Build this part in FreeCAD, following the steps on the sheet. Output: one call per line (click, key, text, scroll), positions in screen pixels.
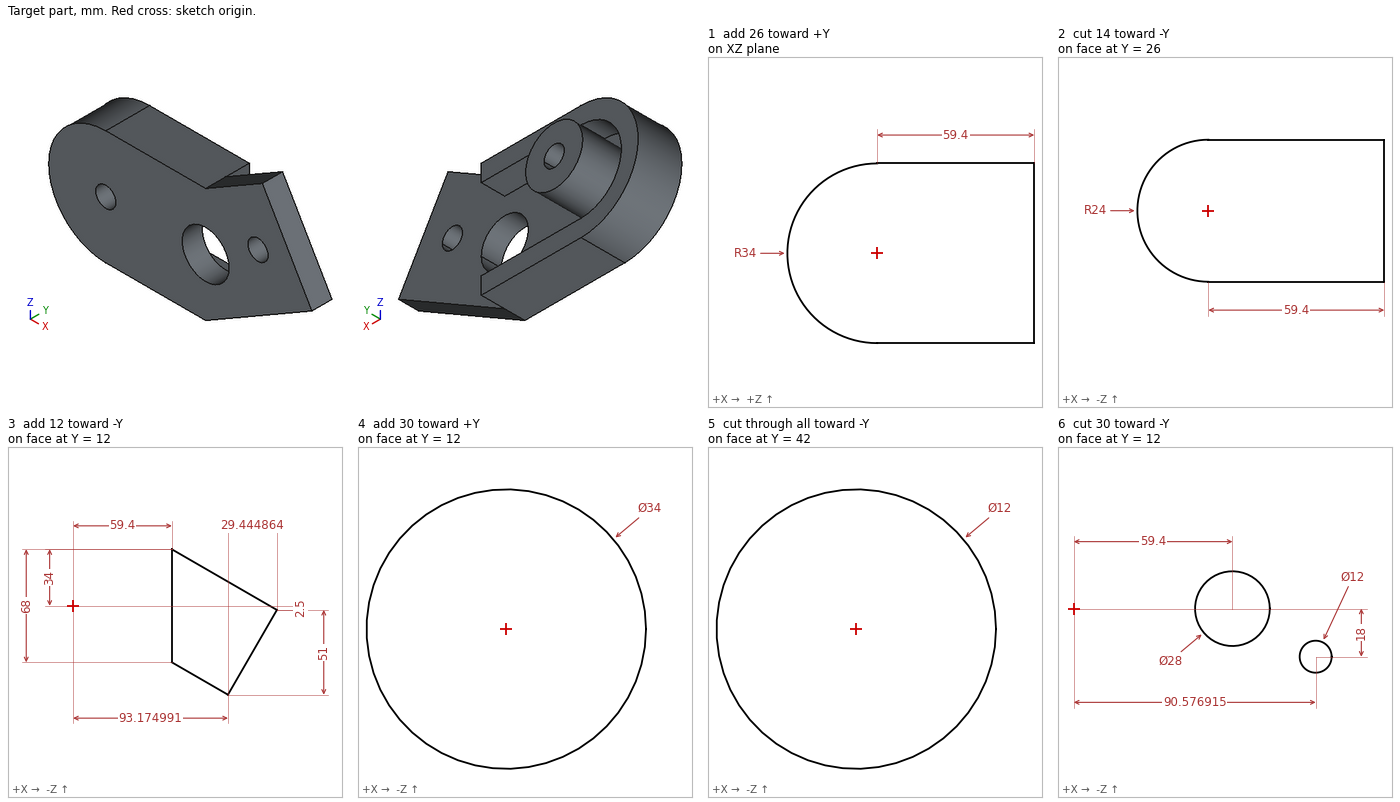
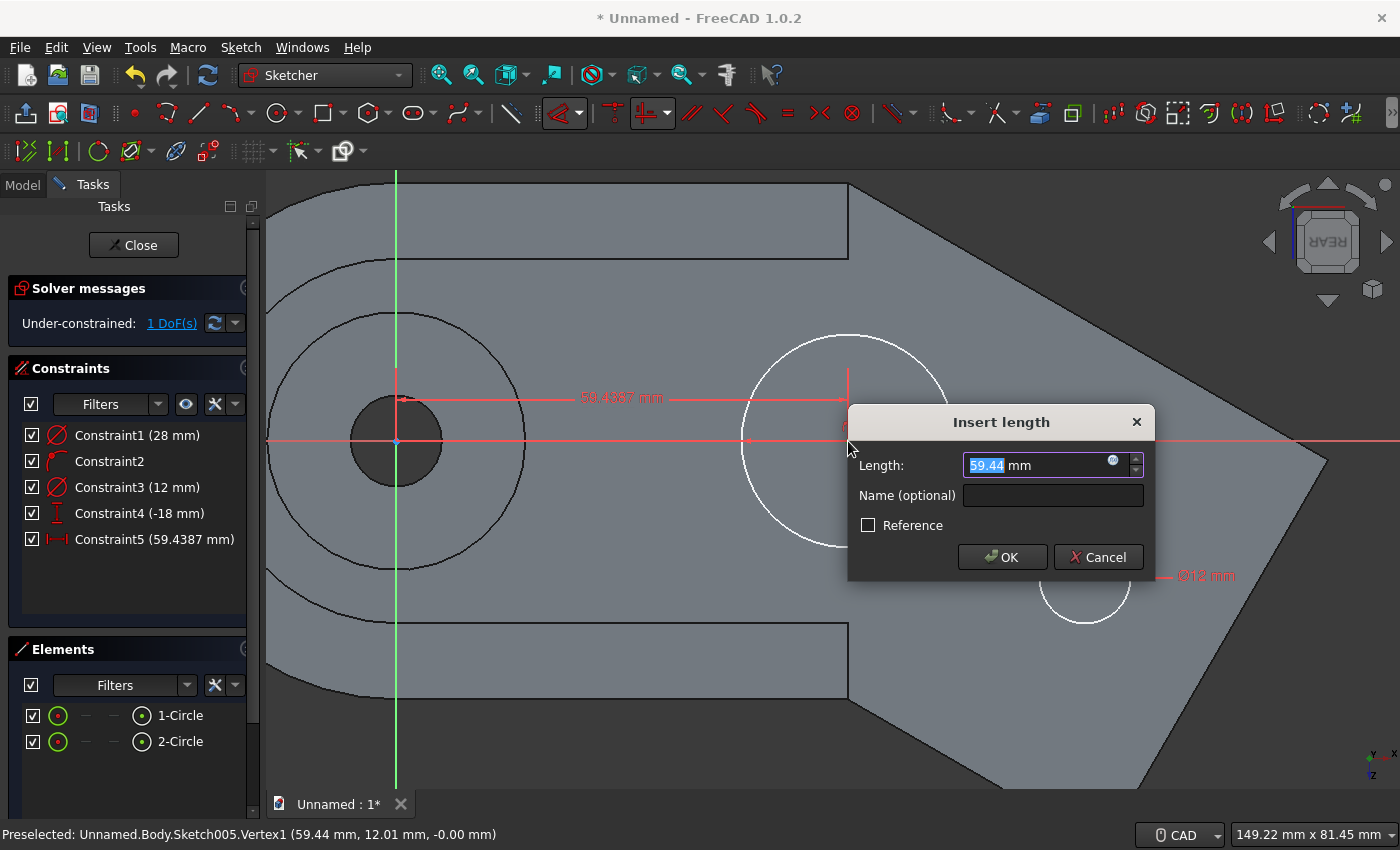
text(59.4)
key(Return)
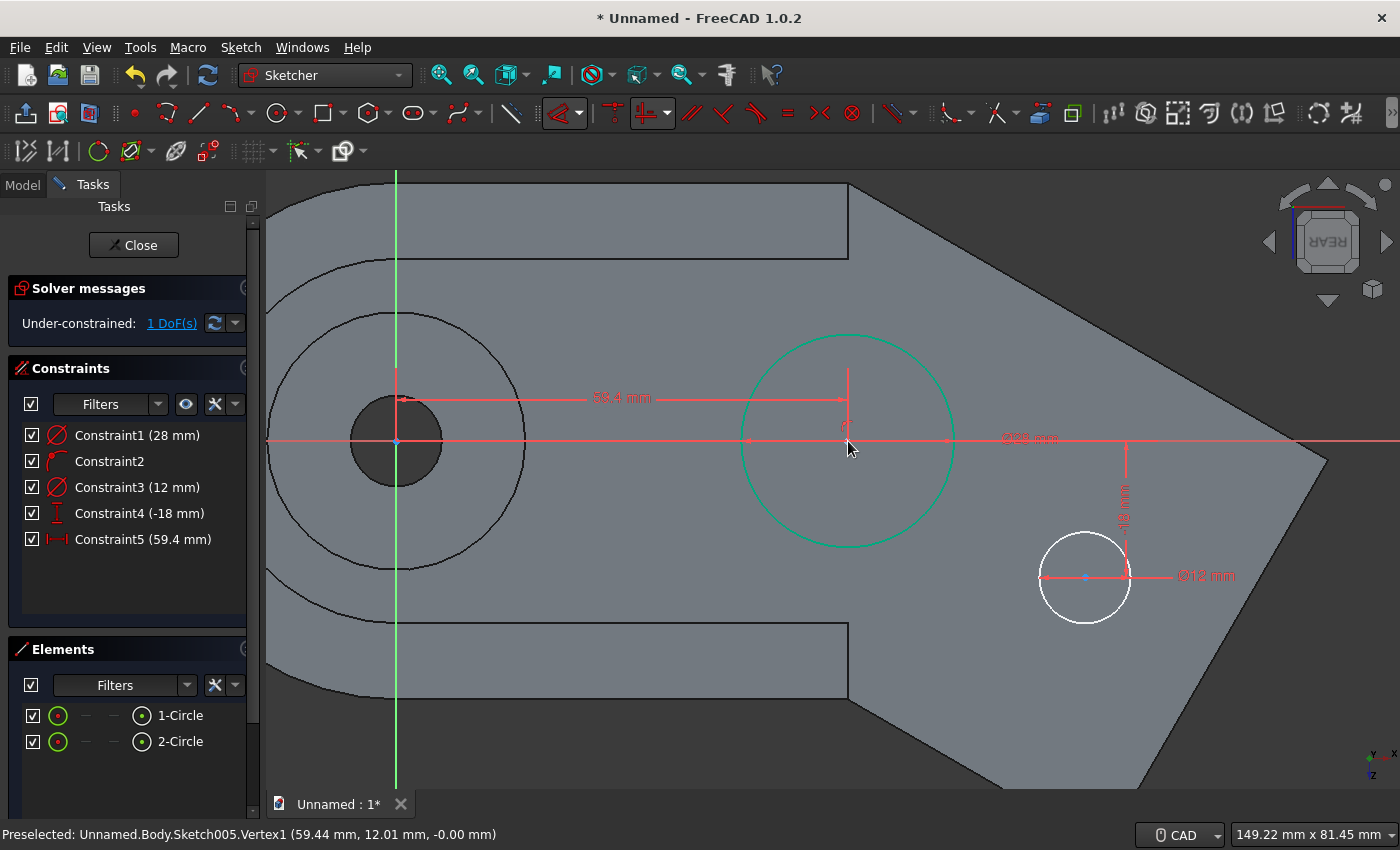
click(1085, 578)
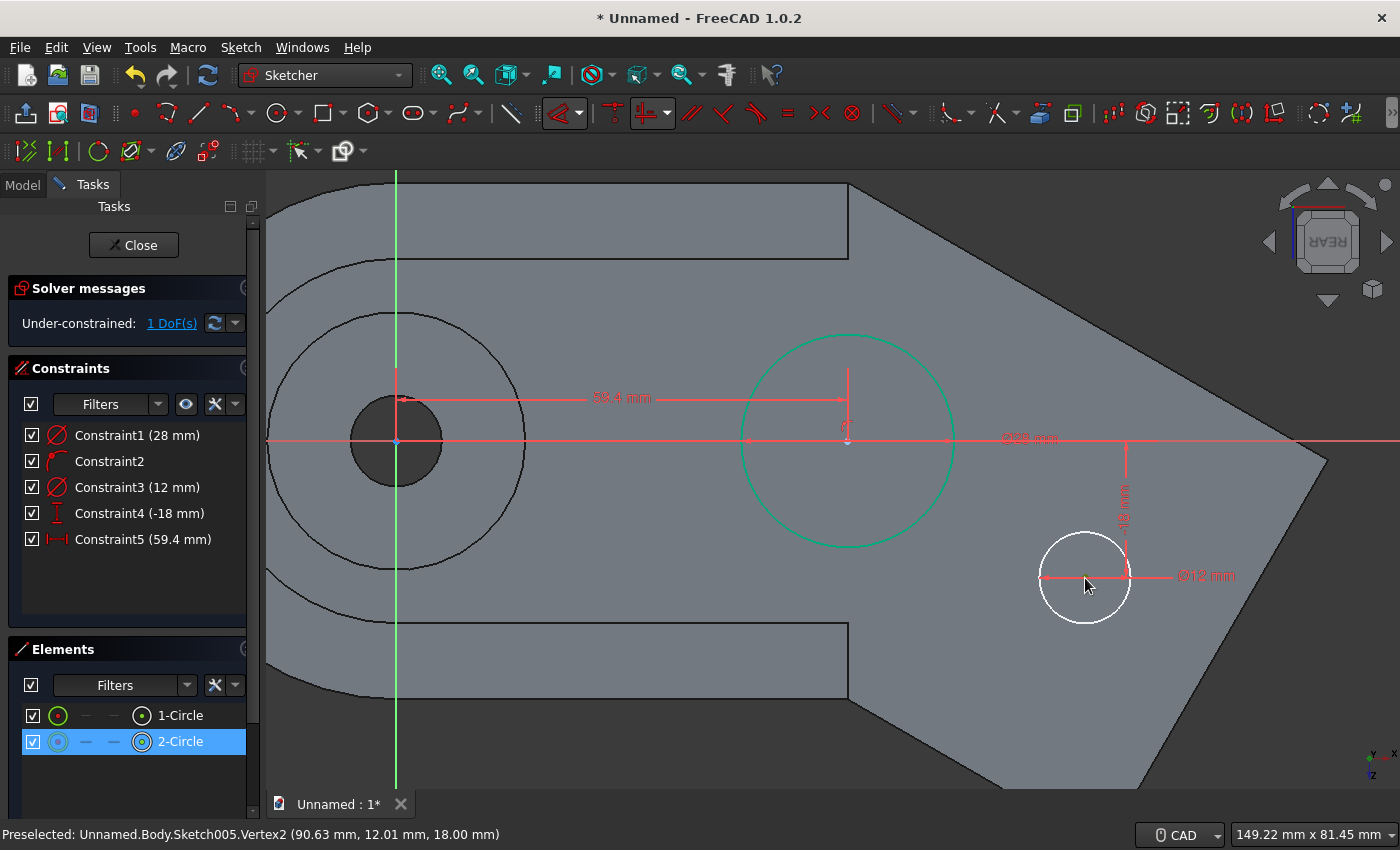
key(l)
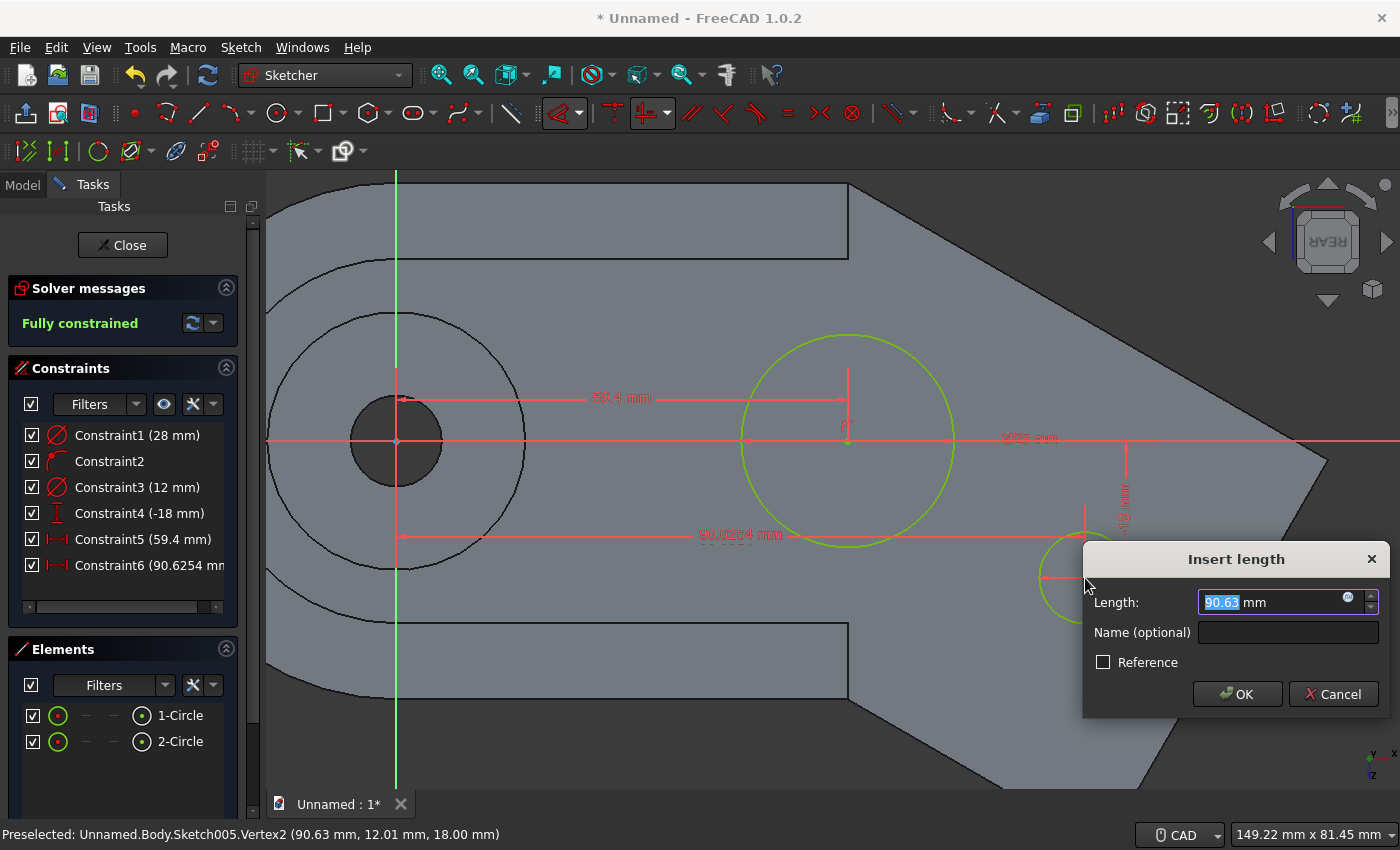
text(90.576915)
key(Return)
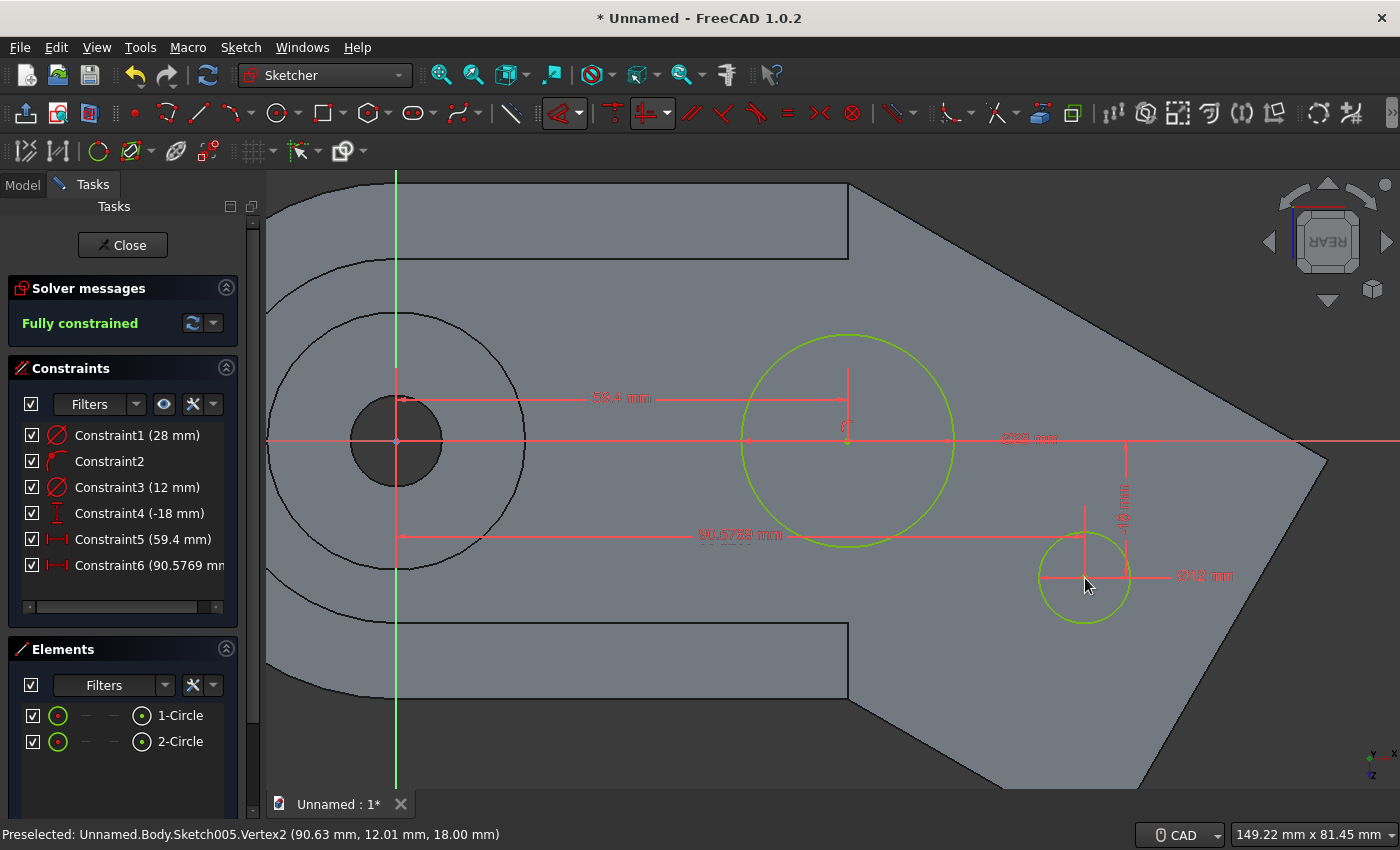
click(123, 245)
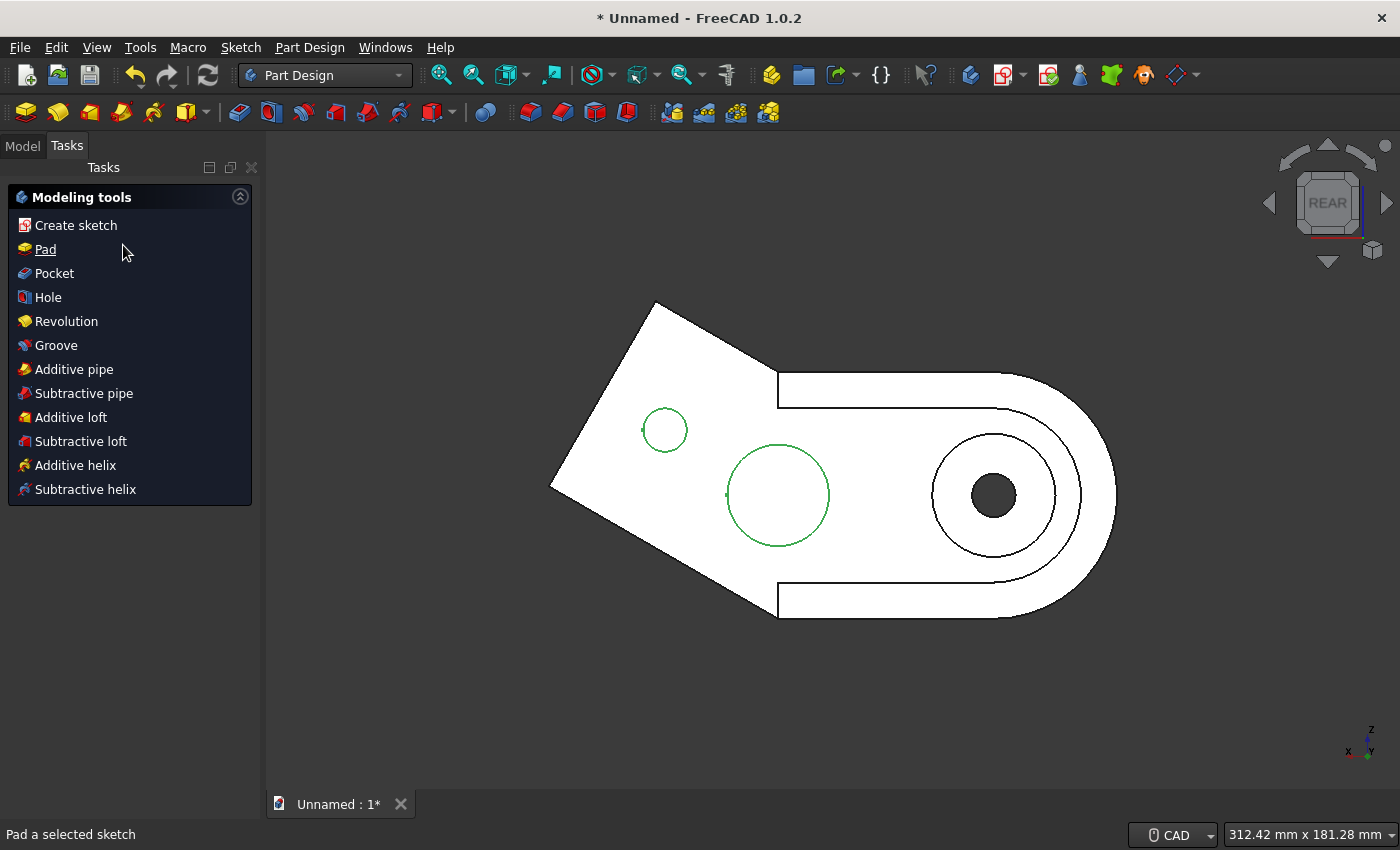
click(240, 112)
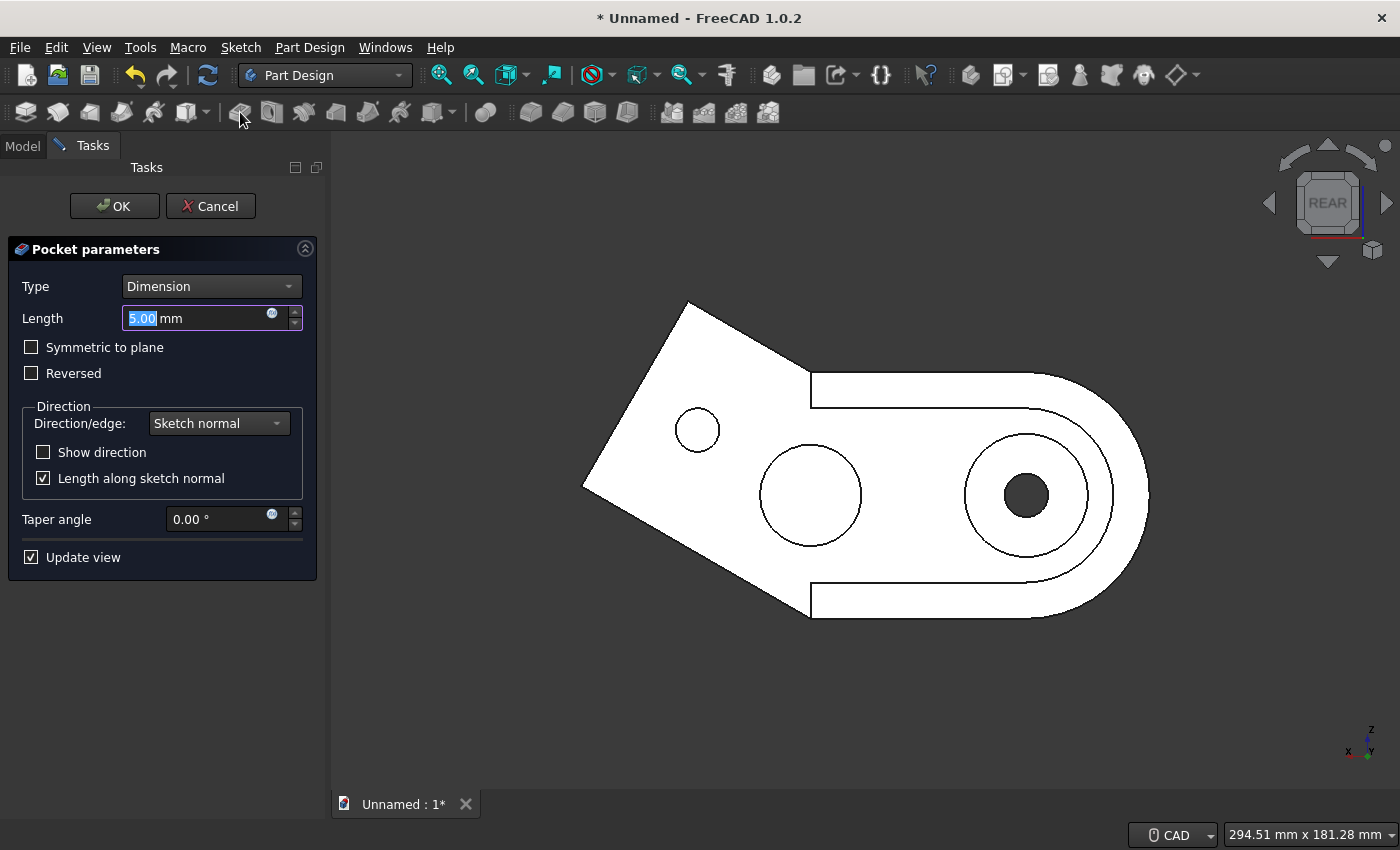
text(30)
key(Tab)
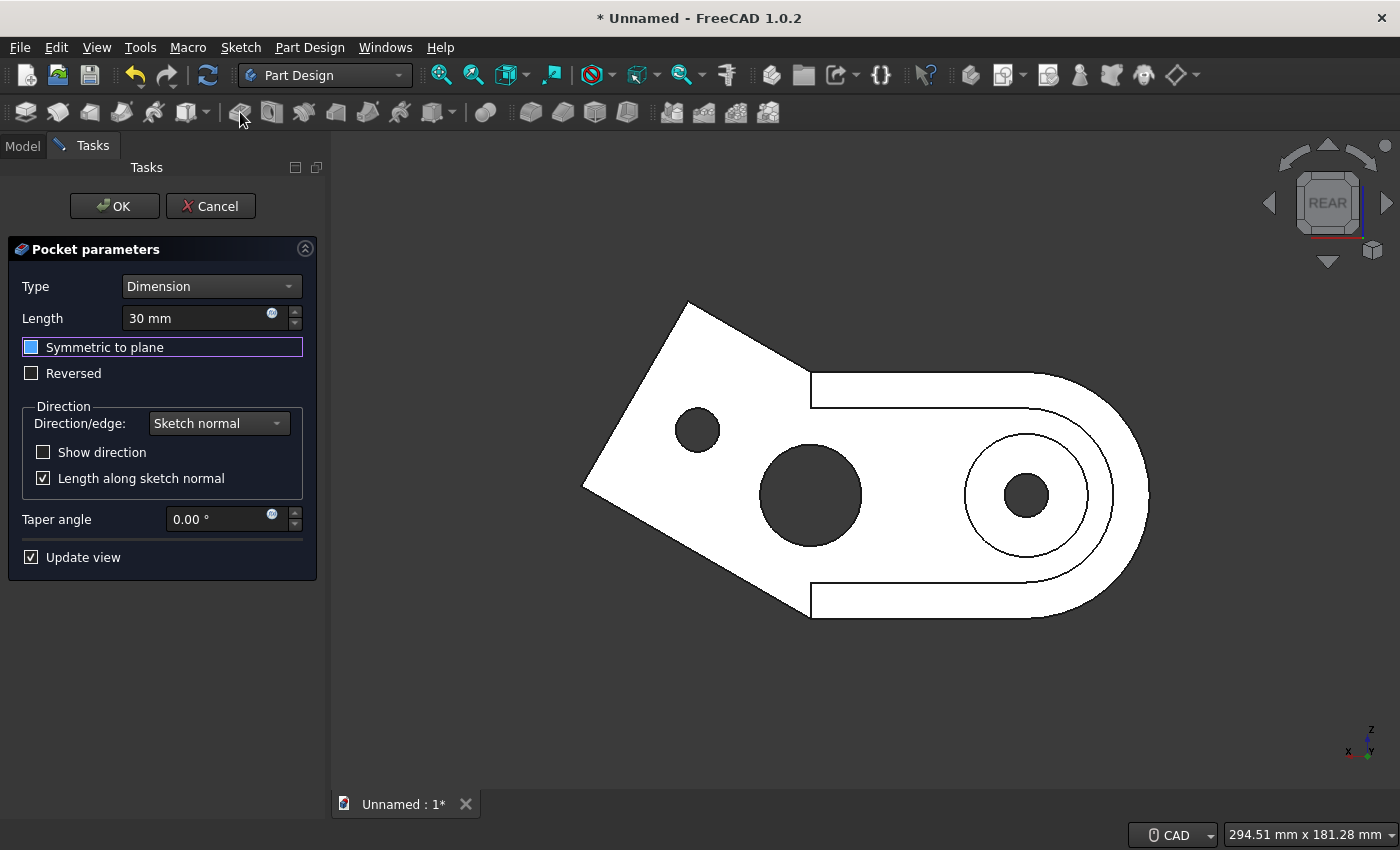
click(115, 206)